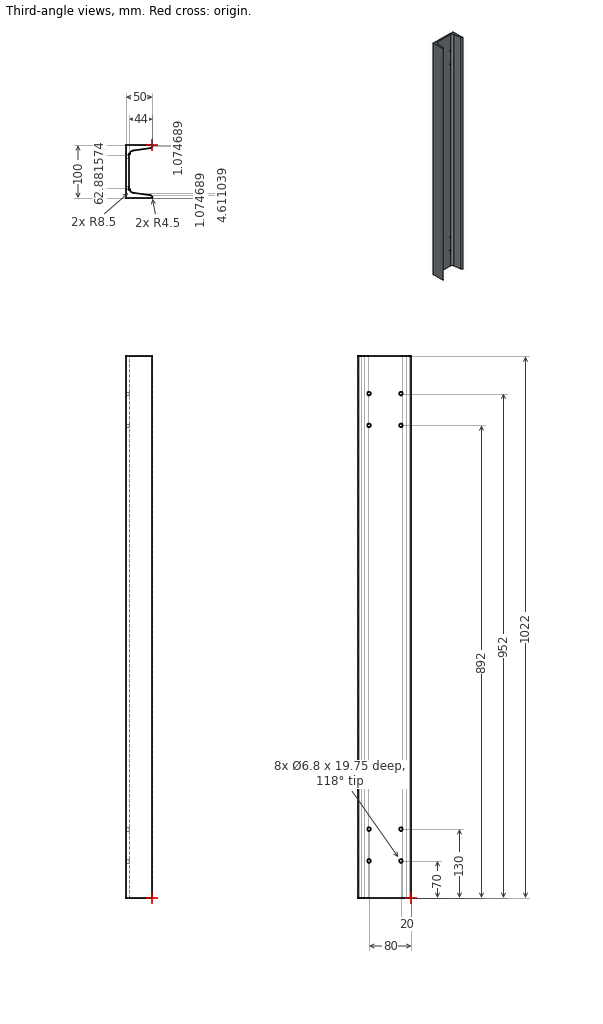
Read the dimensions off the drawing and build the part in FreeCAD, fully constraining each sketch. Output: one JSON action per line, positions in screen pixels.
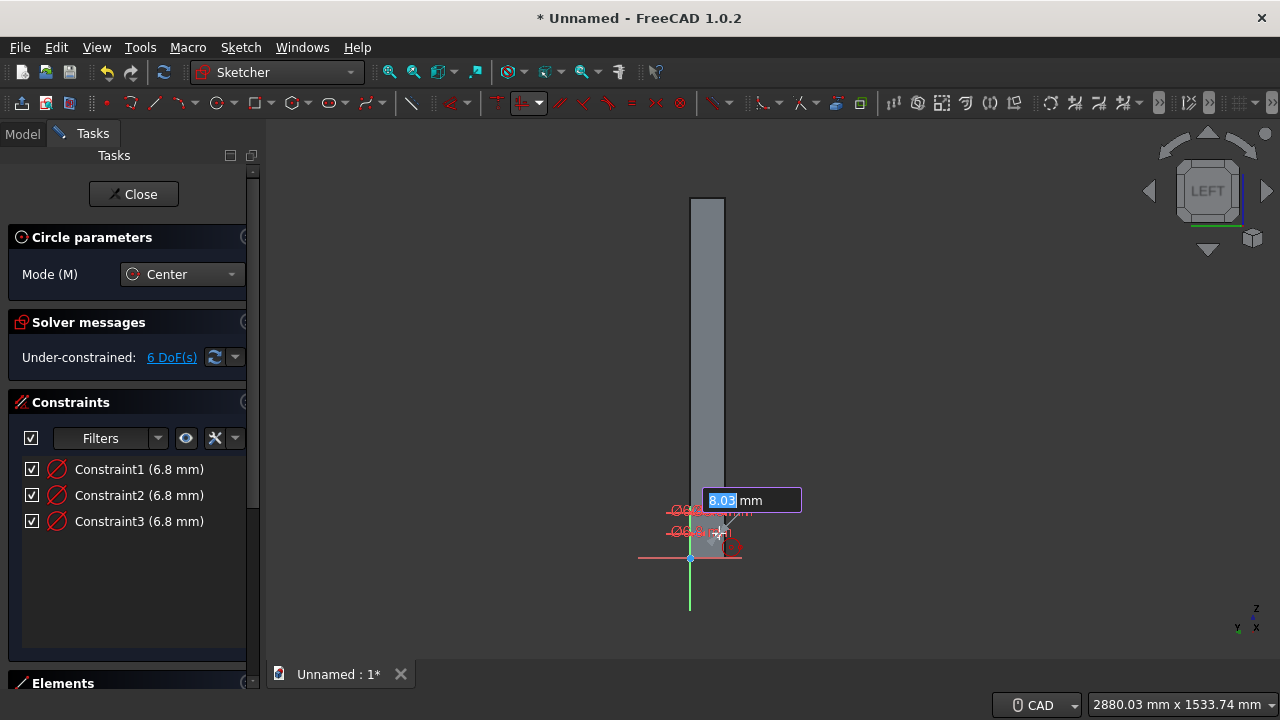
{"action": "type", "text": "6.8"}
{"action": "key", "text": "Return"}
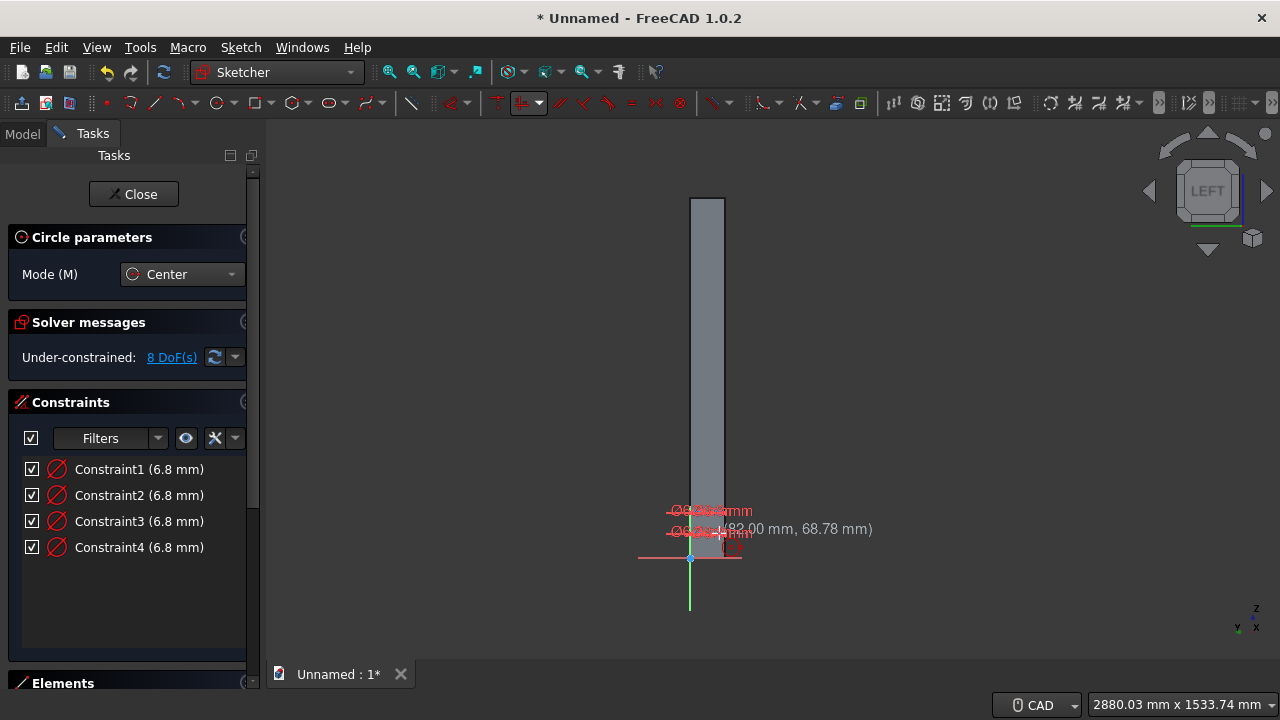
{"action": "scroll", "coordinate": [697, 244], "scroll_direction": "up", "scroll_amount": 15}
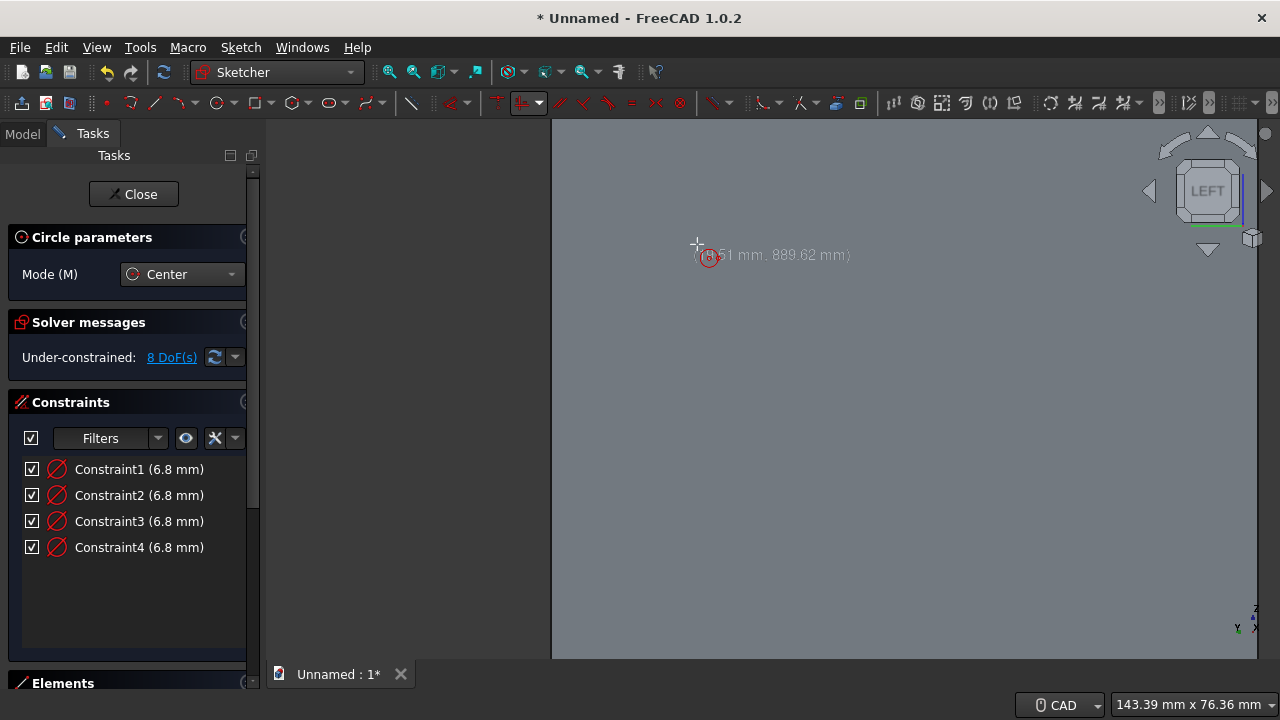
{"action": "scroll", "coordinate": [697, 243], "scroll_direction": "down", "scroll_amount": 15}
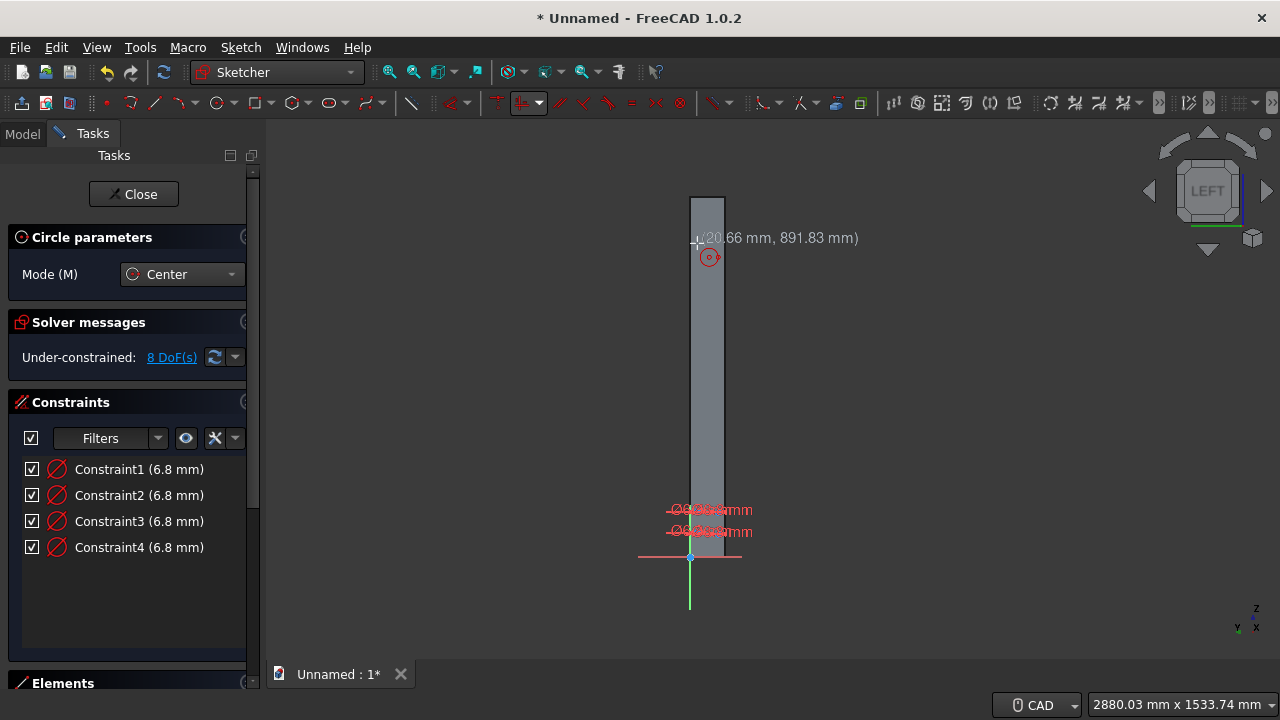
{"action": "scroll", "coordinate": [697, 243], "scroll_direction": "up", "scroll_amount": 5}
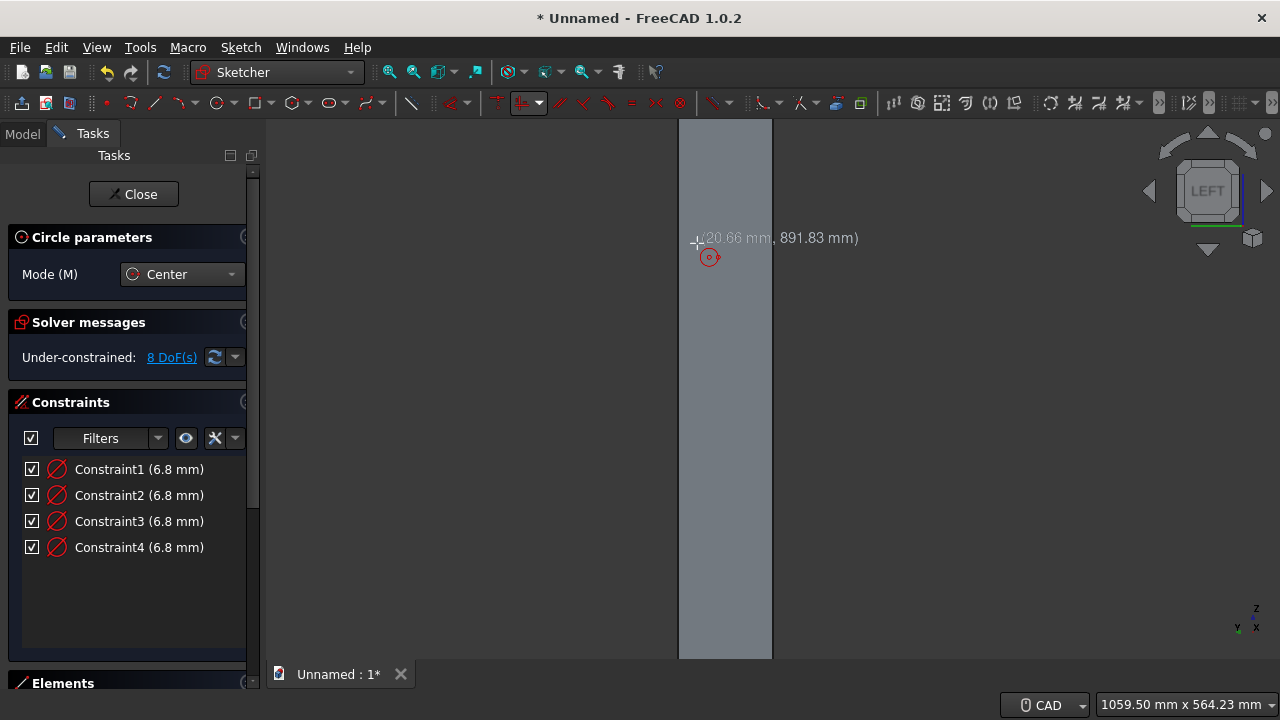
{"action": "left_click", "coordinate": [697, 243]}
{"action": "mouse_move", "coordinate": [699, 241]}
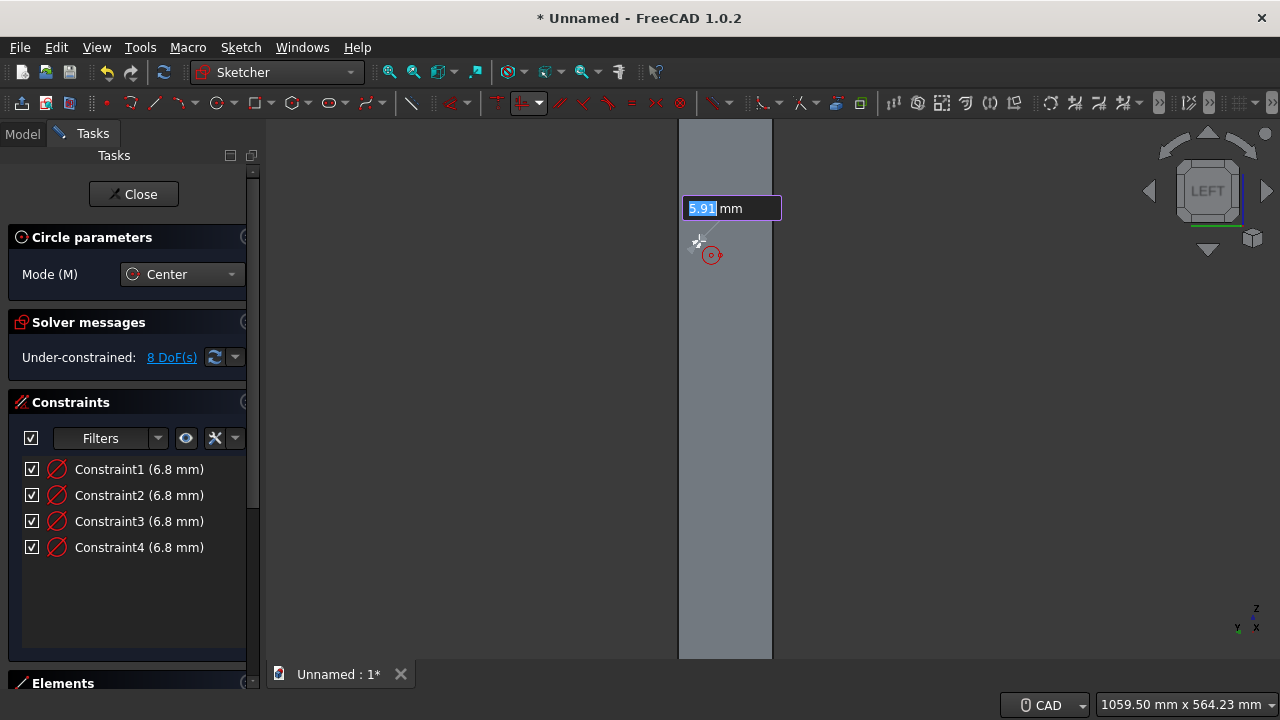
{"action": "type", "text": "6.8"}
{"action": "key", "text": "Return"}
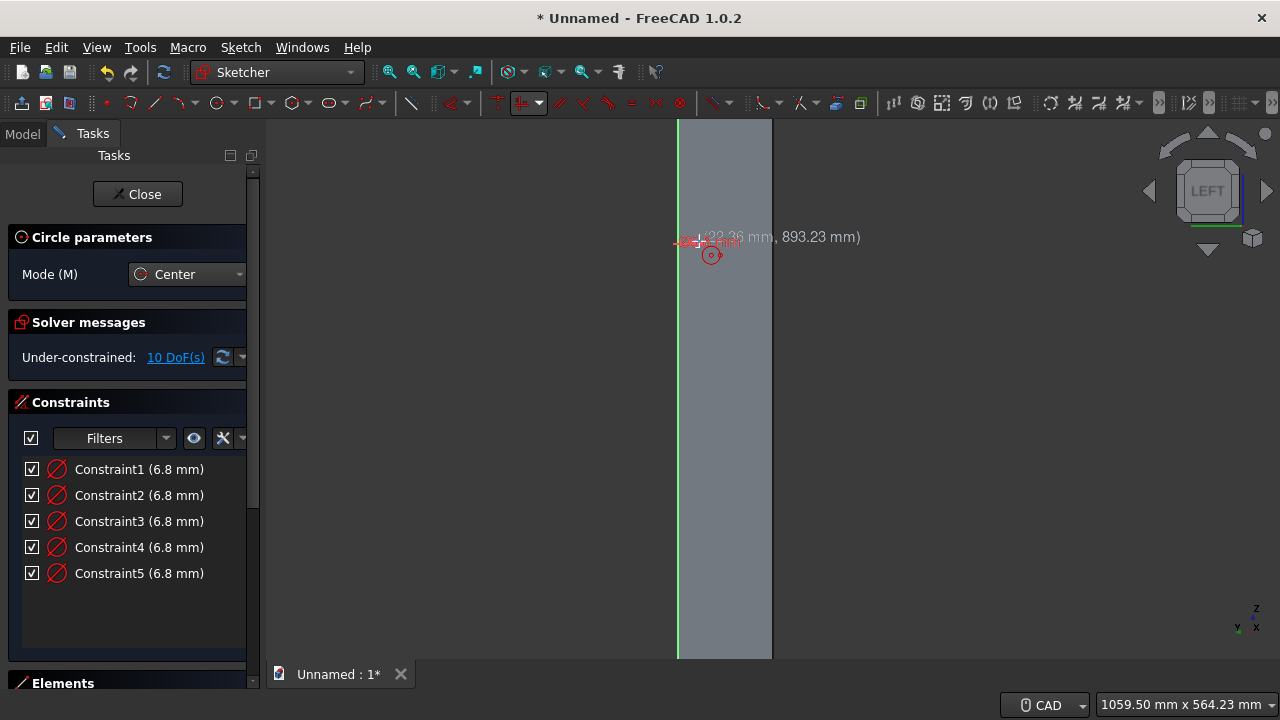
{"action": "scroll", "coordinate": [697, 186], "scroll_direction": "up", "scroll_amount": 10}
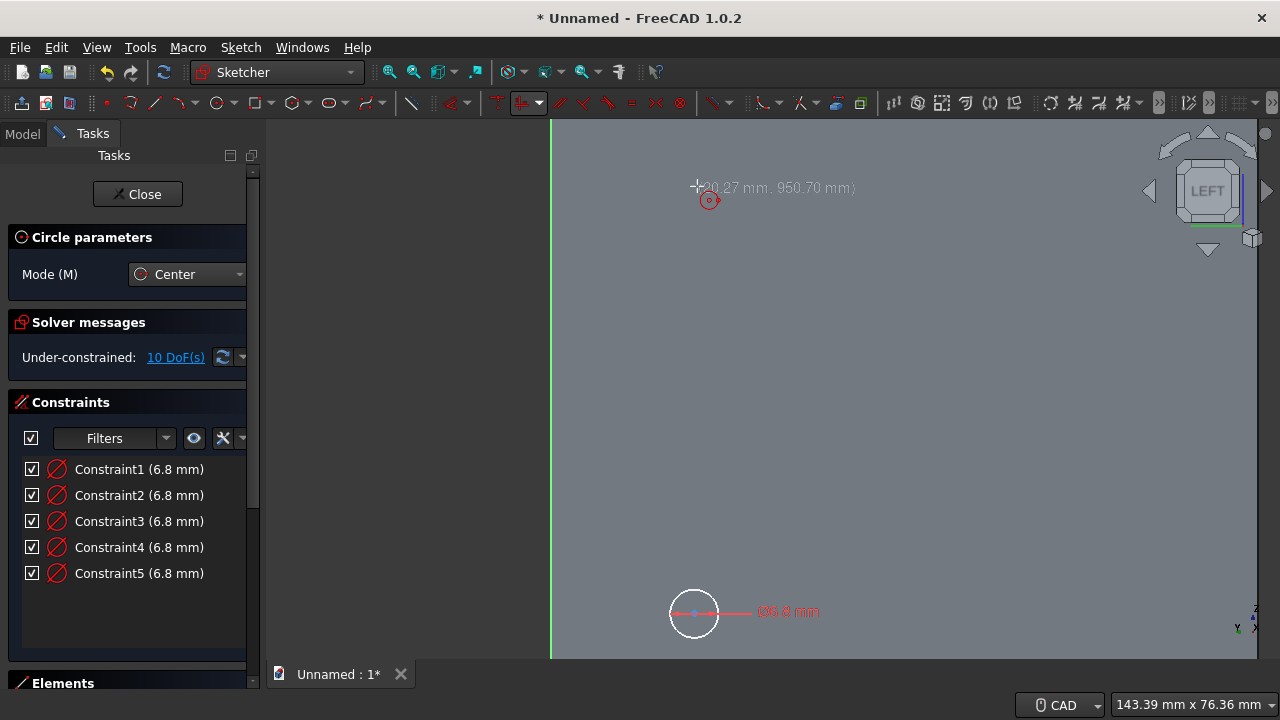
{"action": "scroll", "coordinate": [697, 224], "scroll_direction": "down", "scroll_amount": 15}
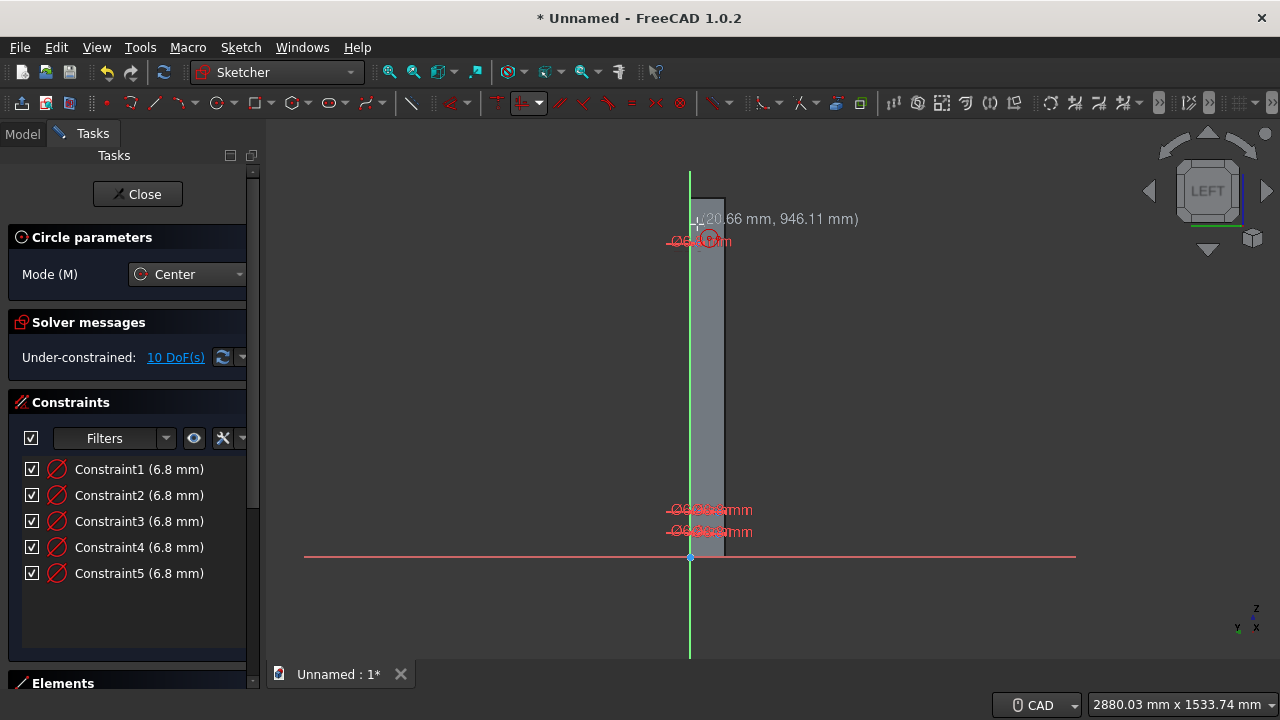
{"action": "scroll", "coordinate": [697, 222], "scroll_direction": "up", "scroll_amount": 5}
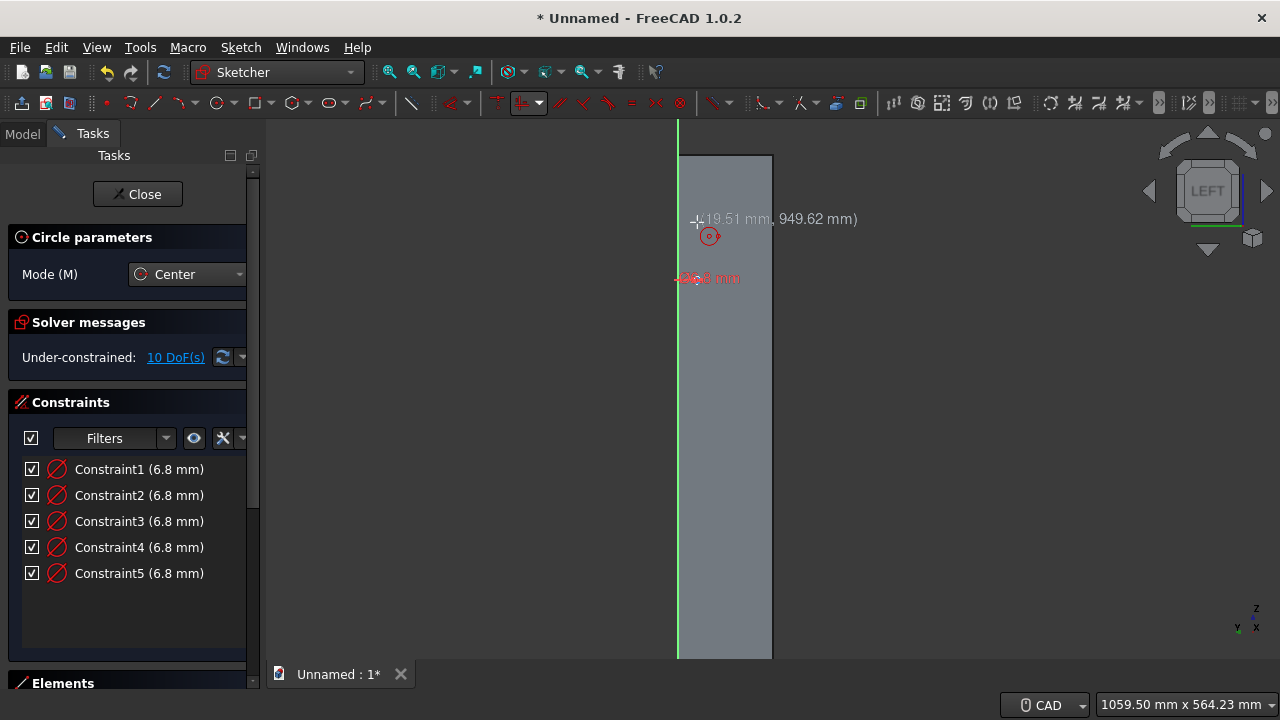
{"action": "left_click", "coordinate": [697, 222]}
{"action": "mouse_move", "coordinate": [699, 220]}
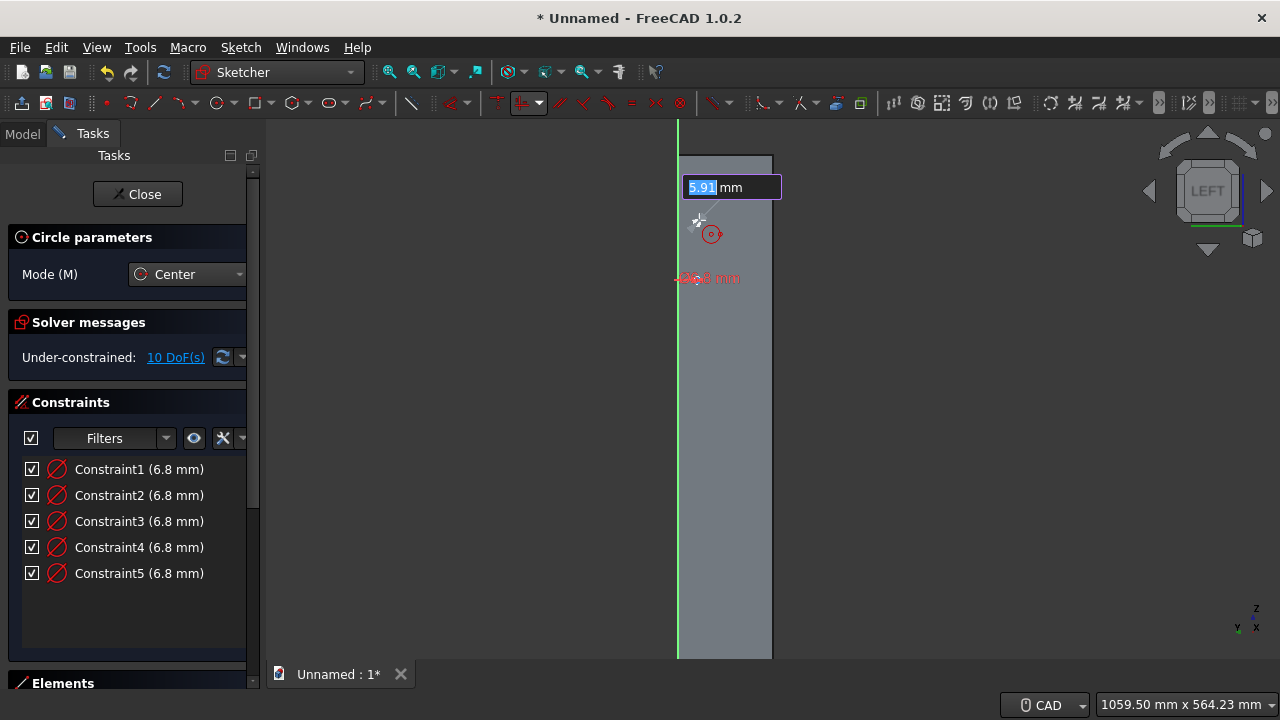
{"action": "type", "text": "6.8"}
{"action": "key", "text": "Return"}